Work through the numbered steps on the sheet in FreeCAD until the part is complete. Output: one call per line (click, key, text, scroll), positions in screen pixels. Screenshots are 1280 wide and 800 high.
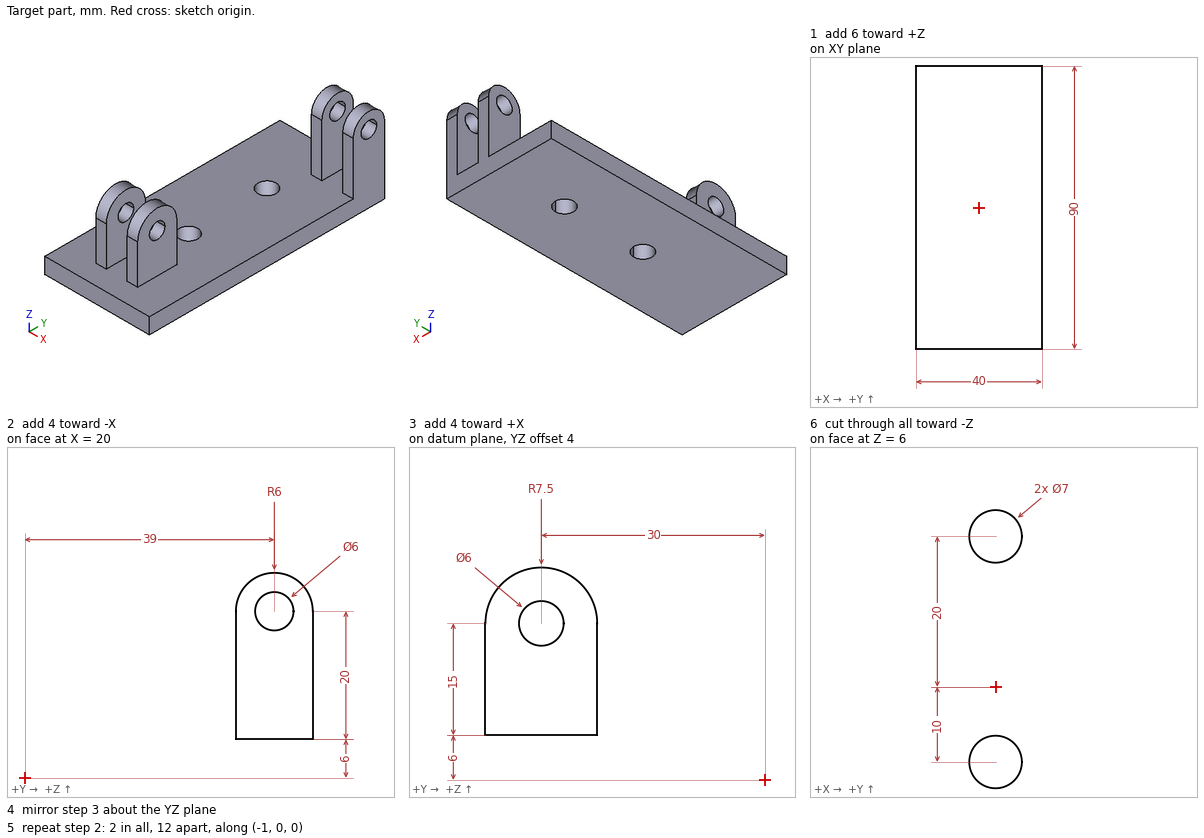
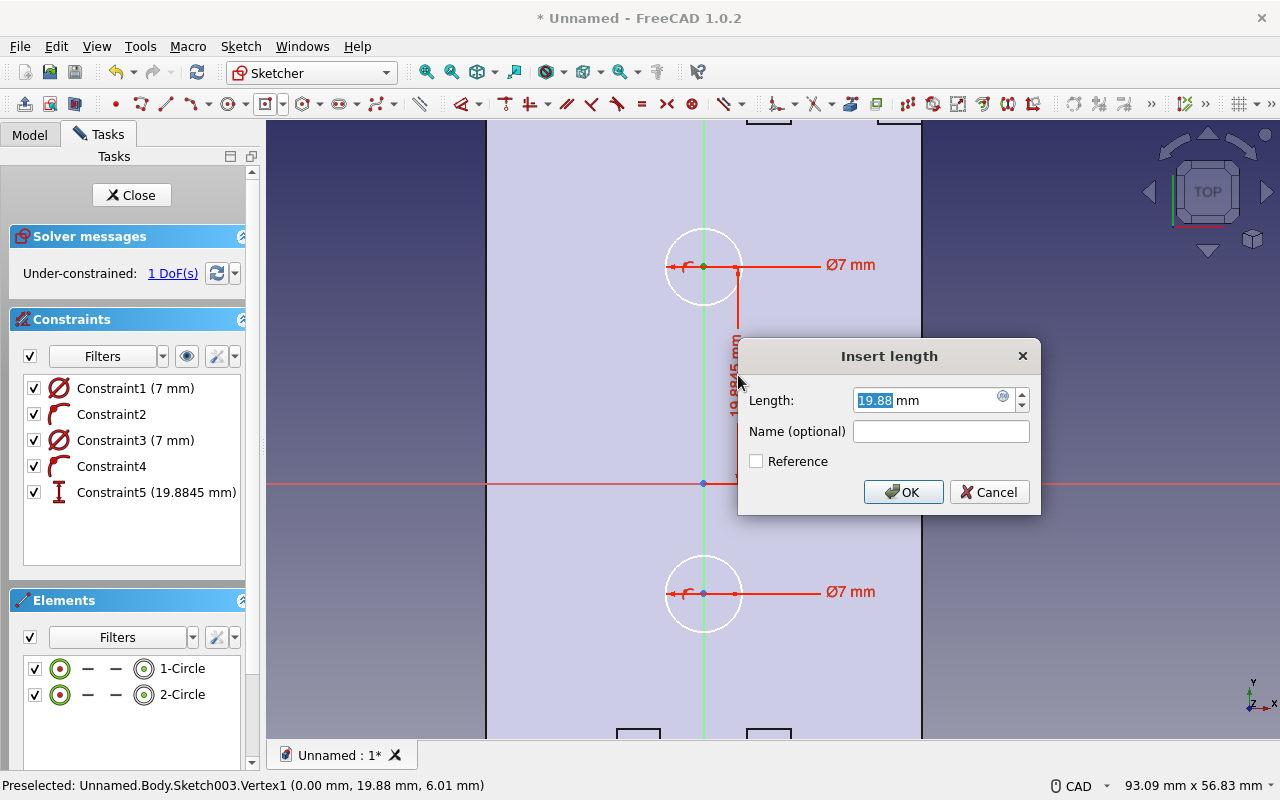
text(20)
key(Return)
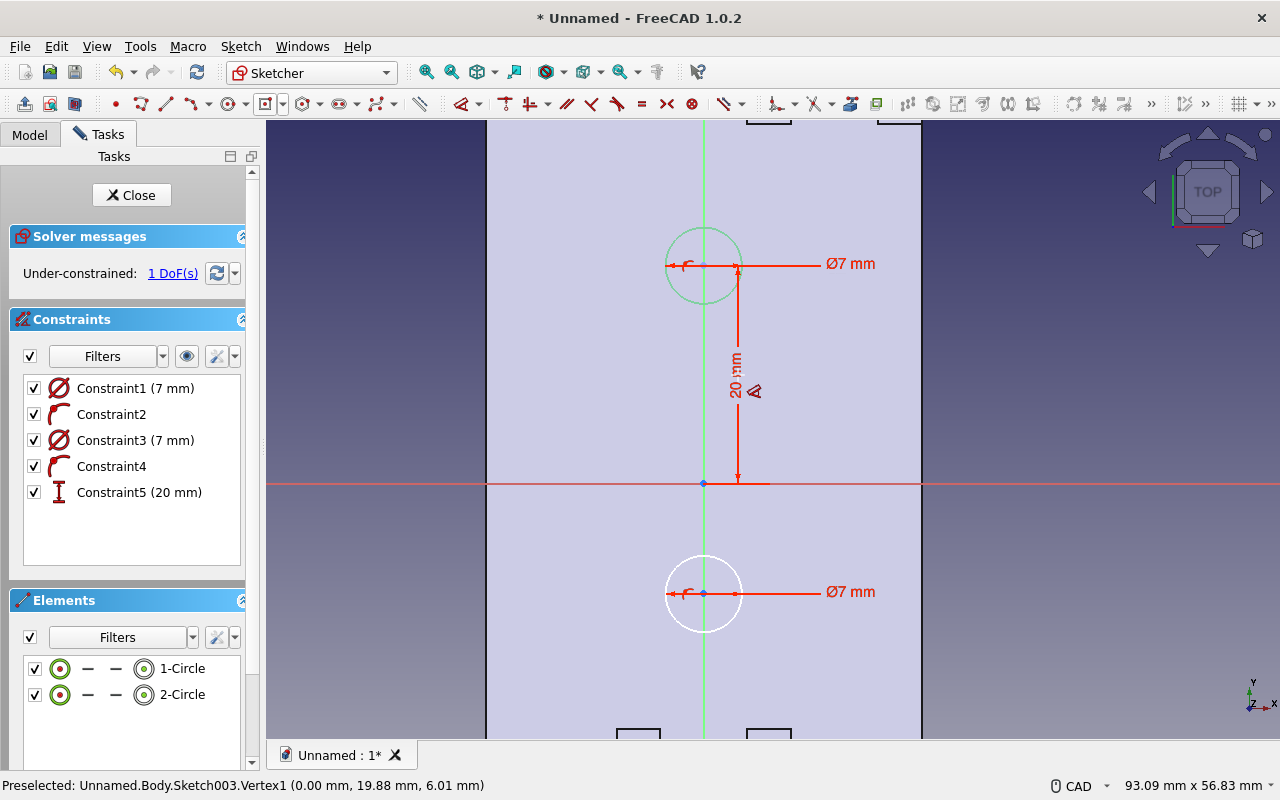
click(704, 594)
click(738, 539)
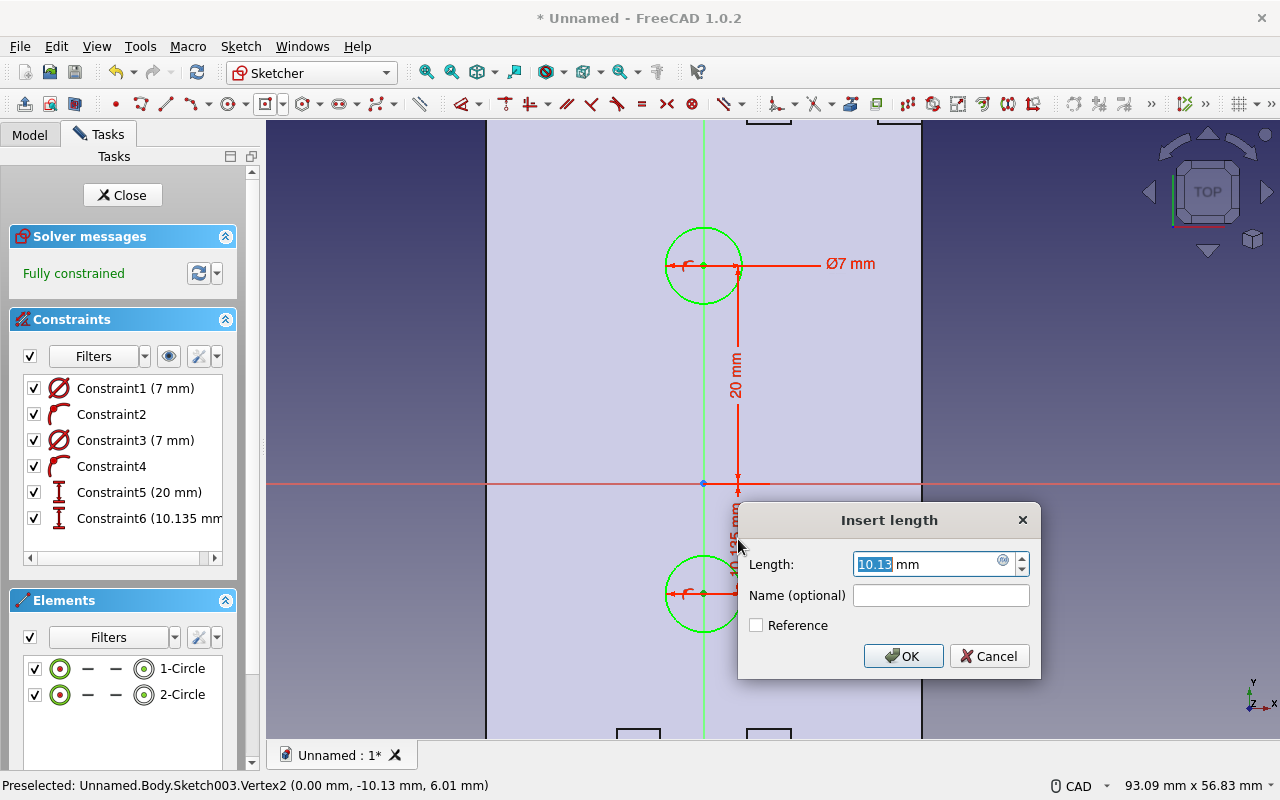
text(10)
key(Return)
key(Escape)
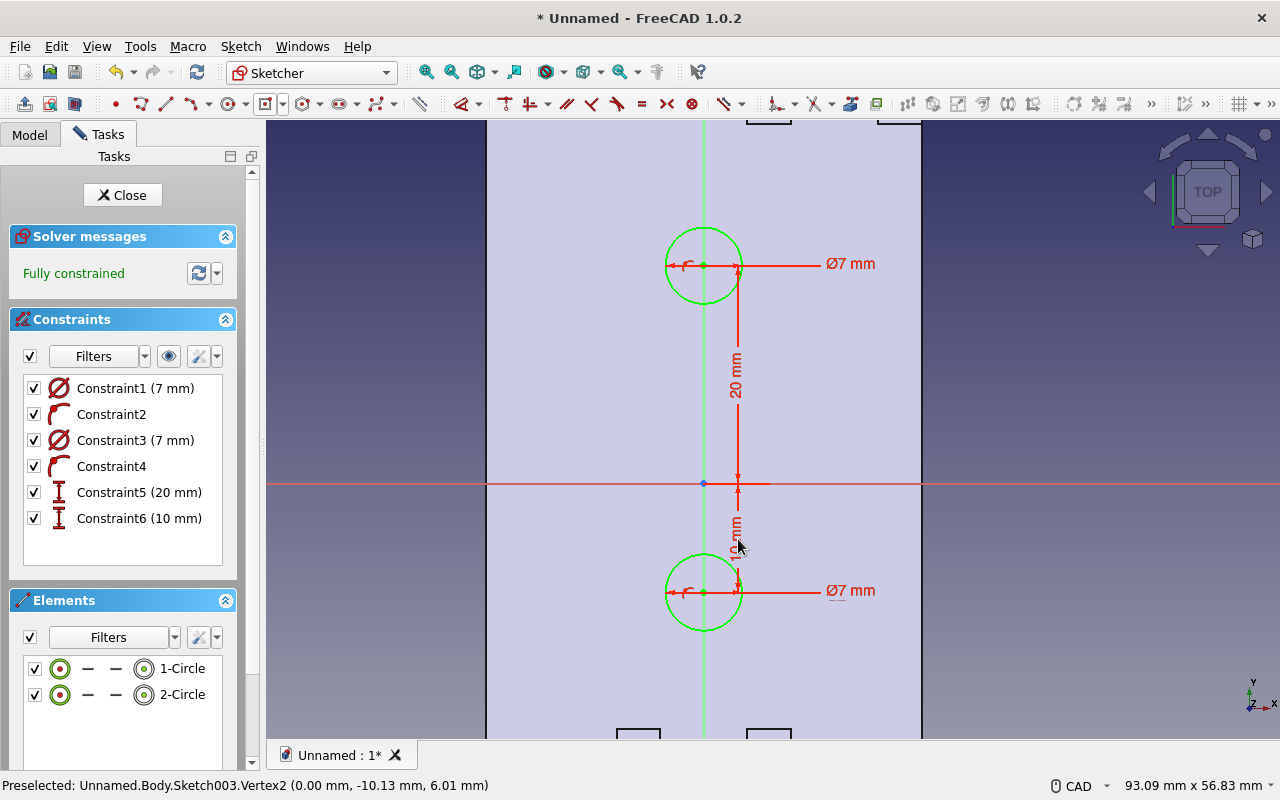
click(123, 195)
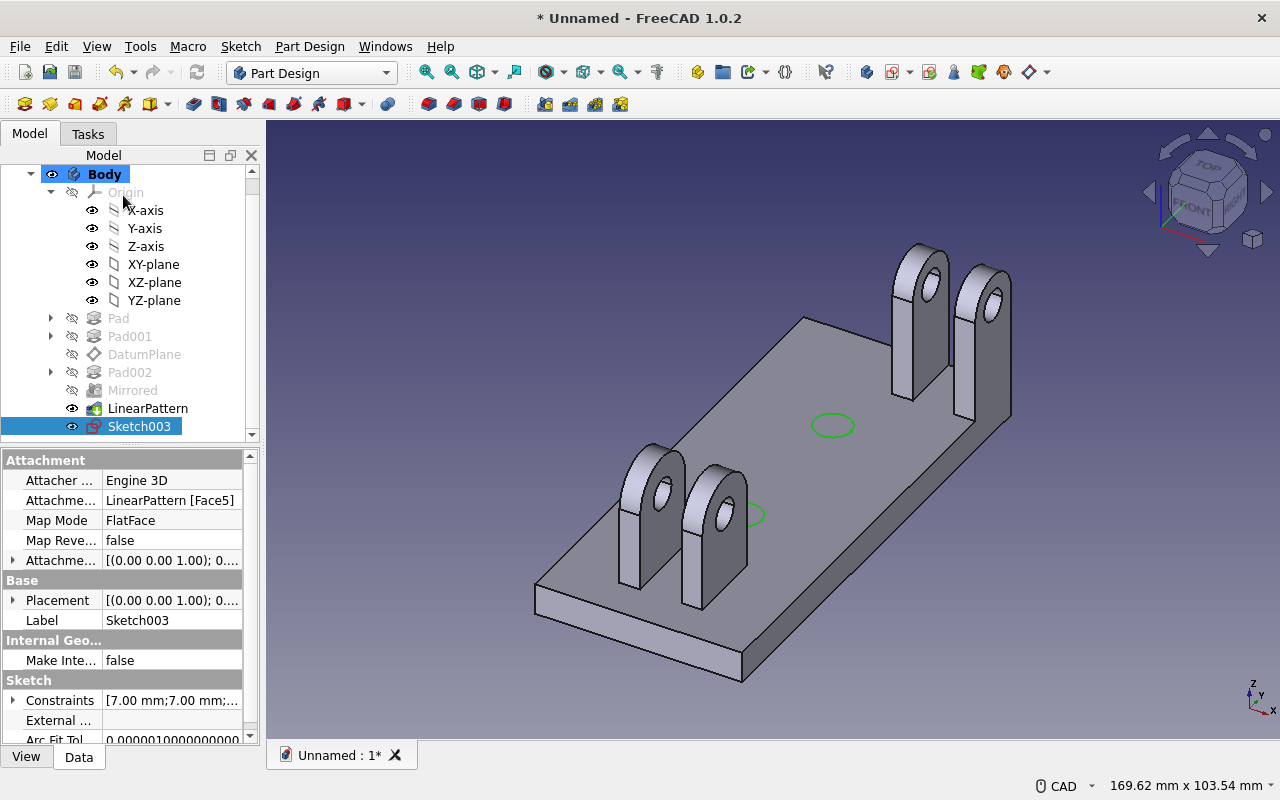
click(194, 104)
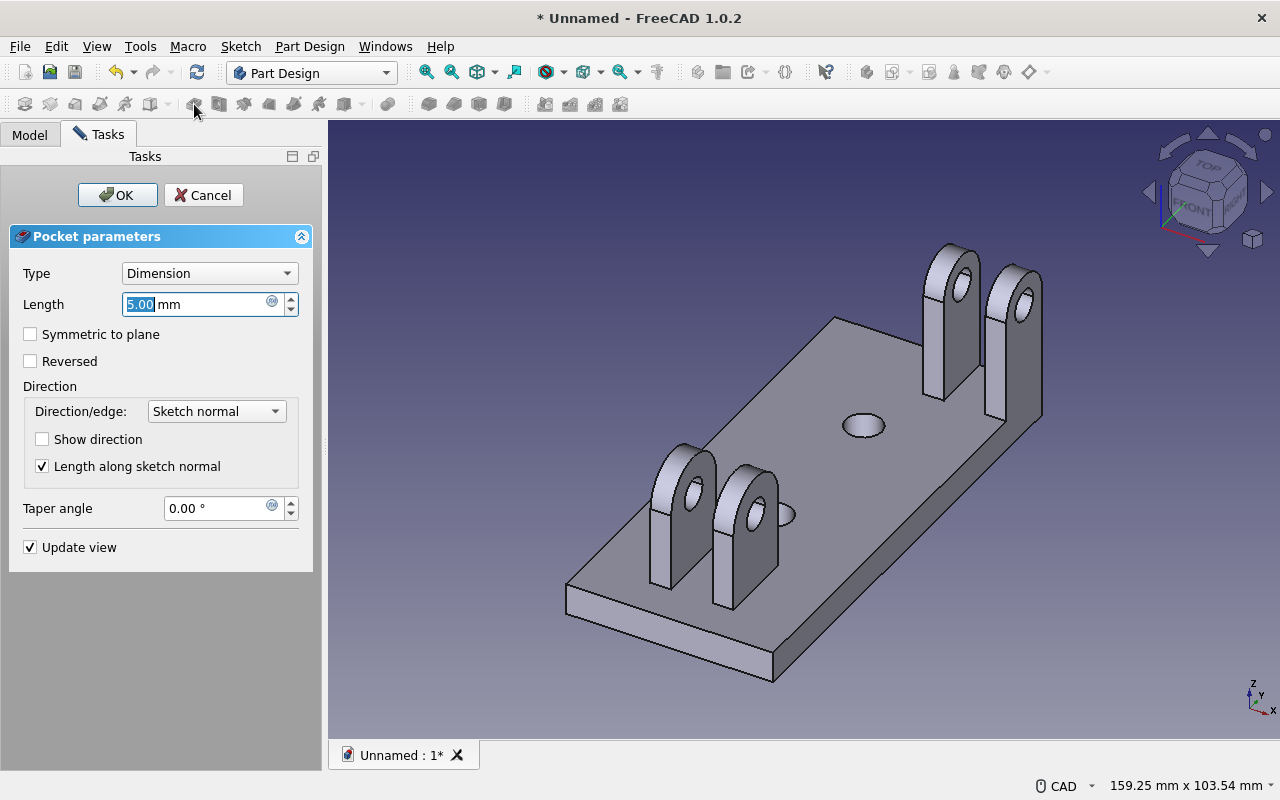
click(210, 274)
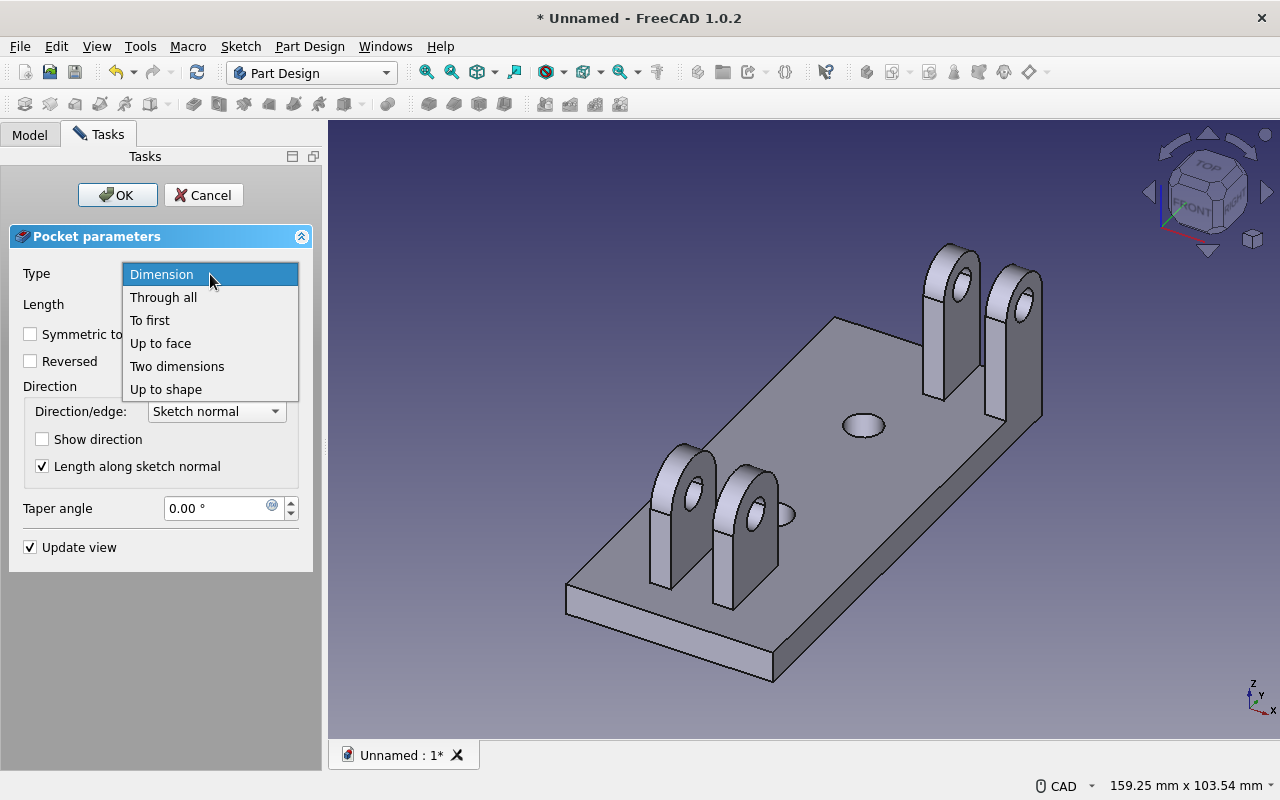
click(208, 298)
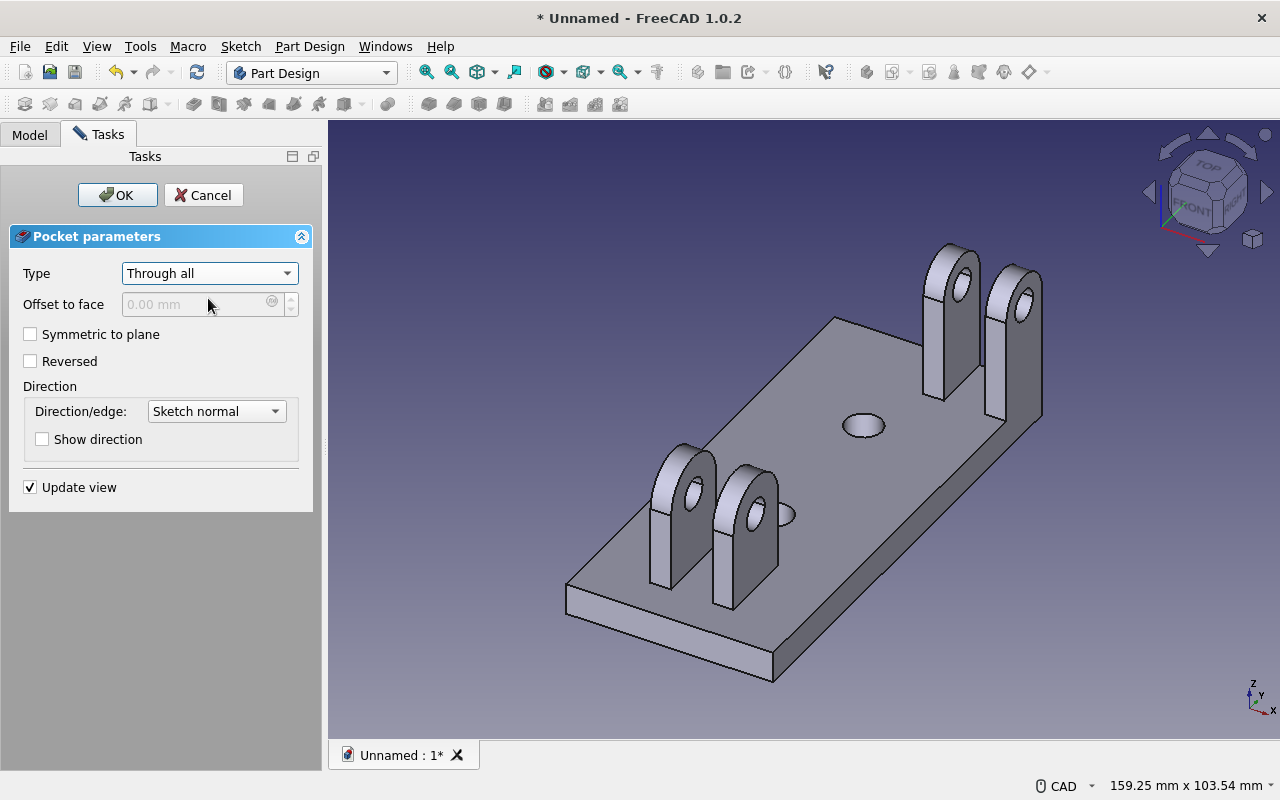
click(118, 195)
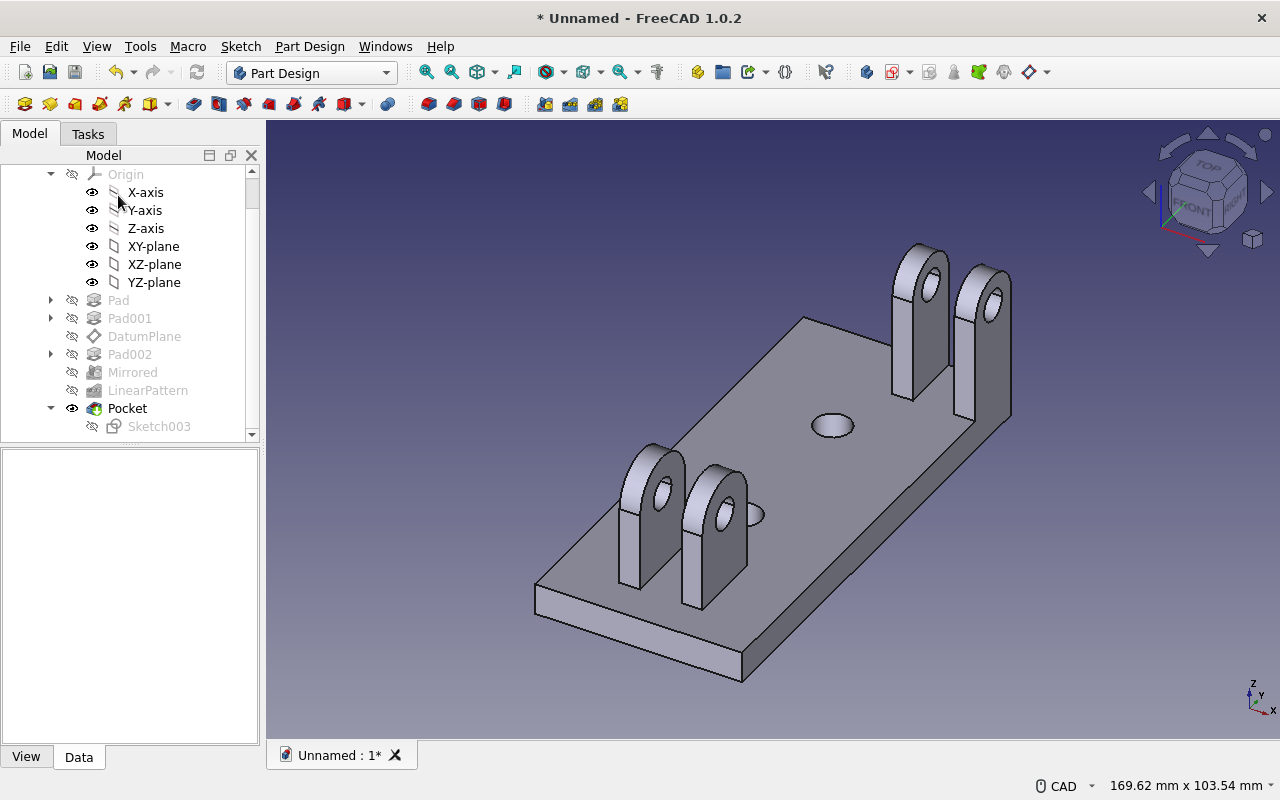
key(0)